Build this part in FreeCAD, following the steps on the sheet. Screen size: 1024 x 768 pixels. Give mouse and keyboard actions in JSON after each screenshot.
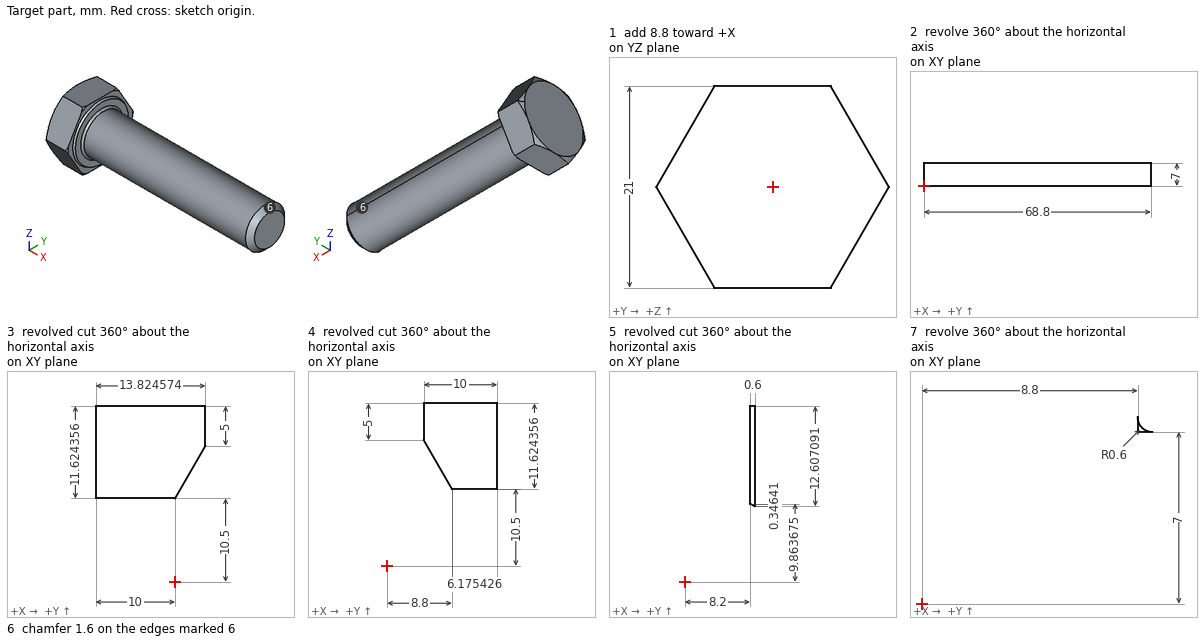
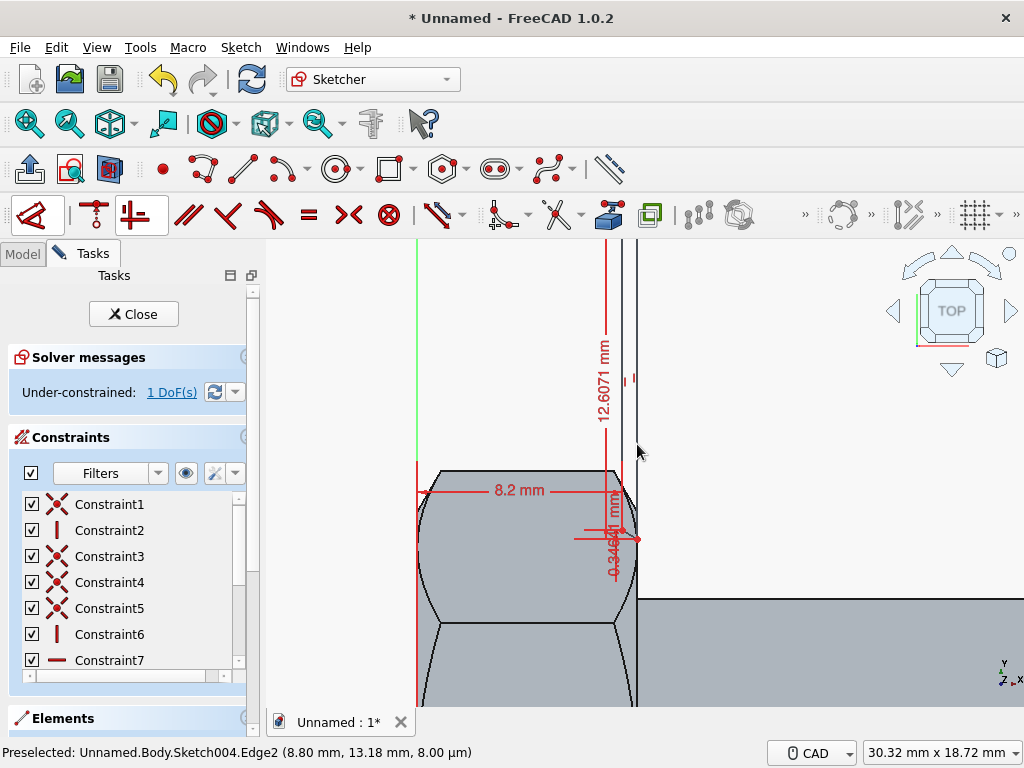
{"action": "left_click", "coordinate": [622, 530]}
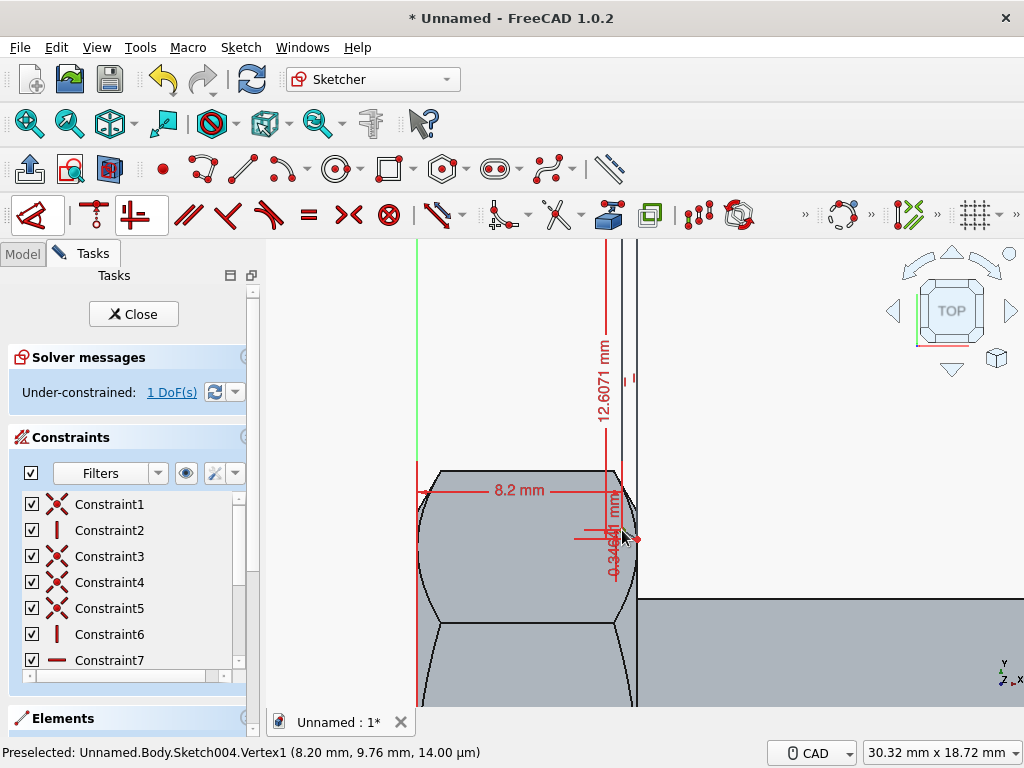
{"action": "key", "text": "i"}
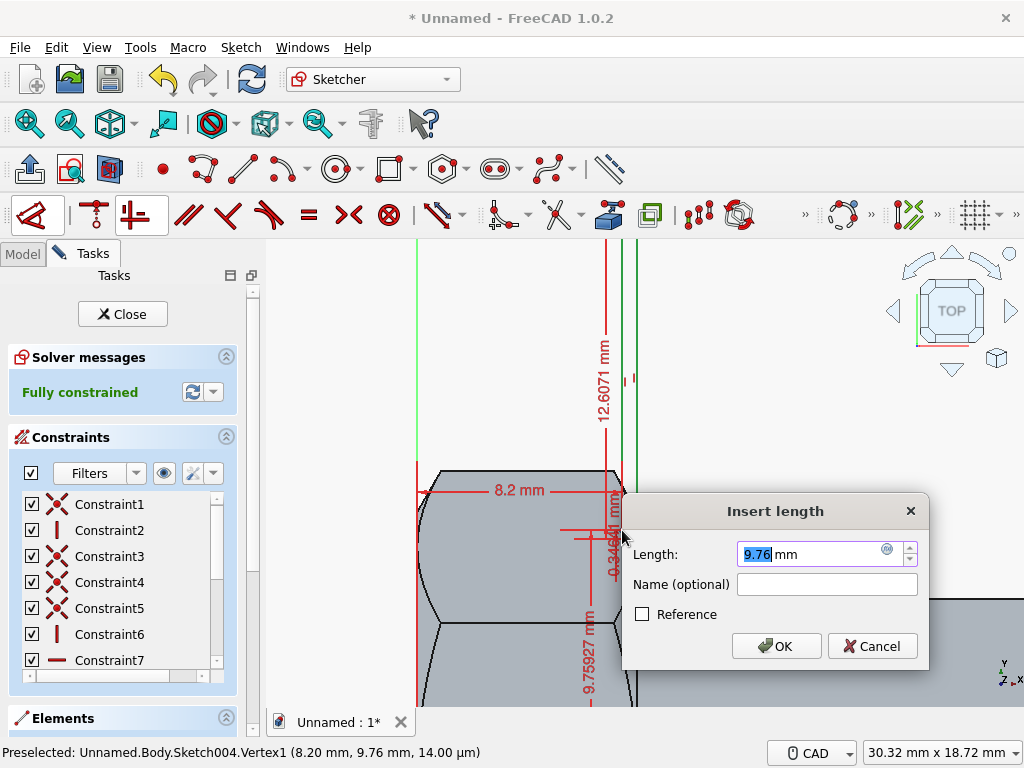
{"action": "type", "text": "9.863675"}
{"action": "key", "text": "Return"}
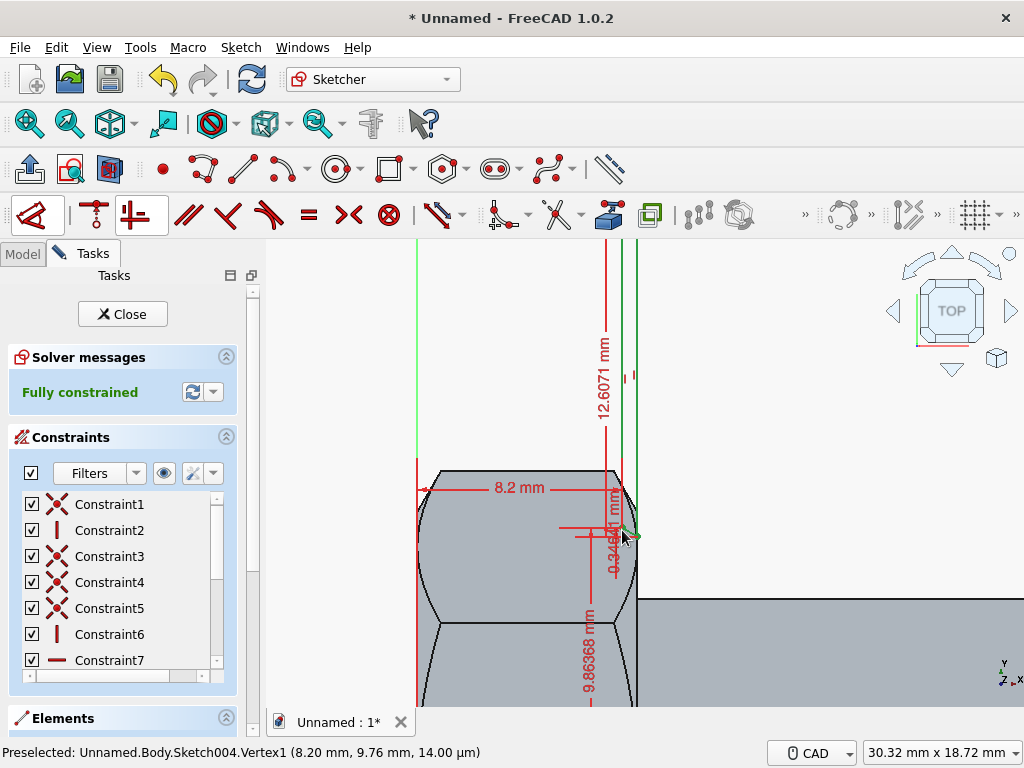
{"action": "left_click", "coordinate": [123, 314]}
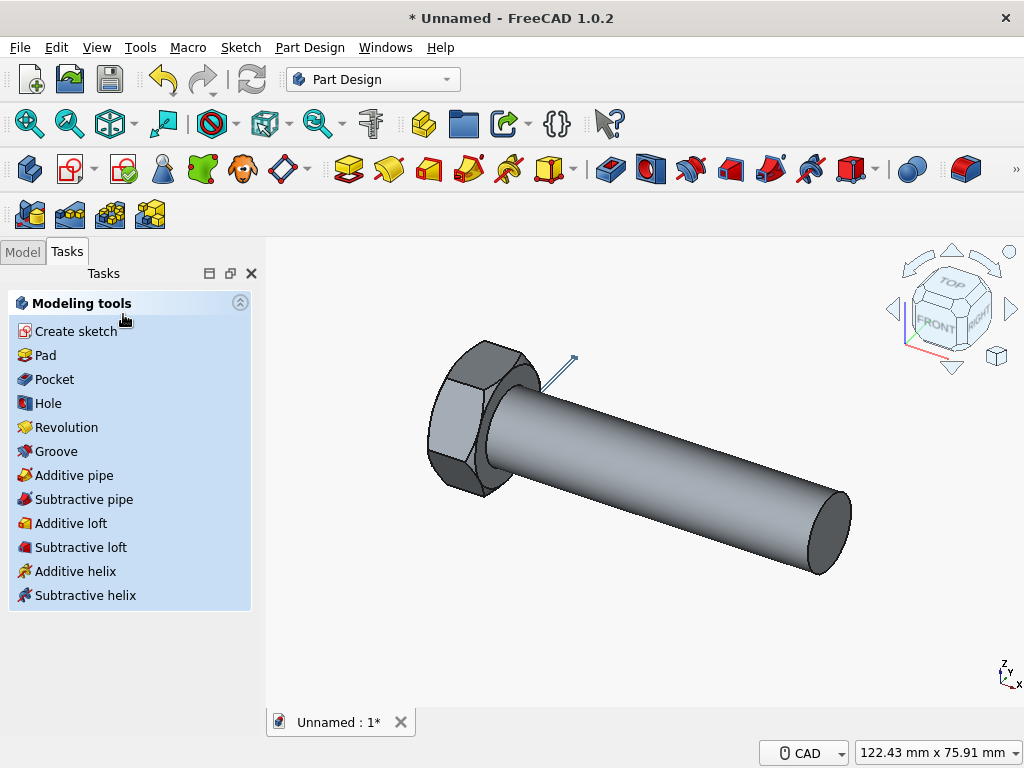
{"action": "left_click", "coordinate": [692, 170]}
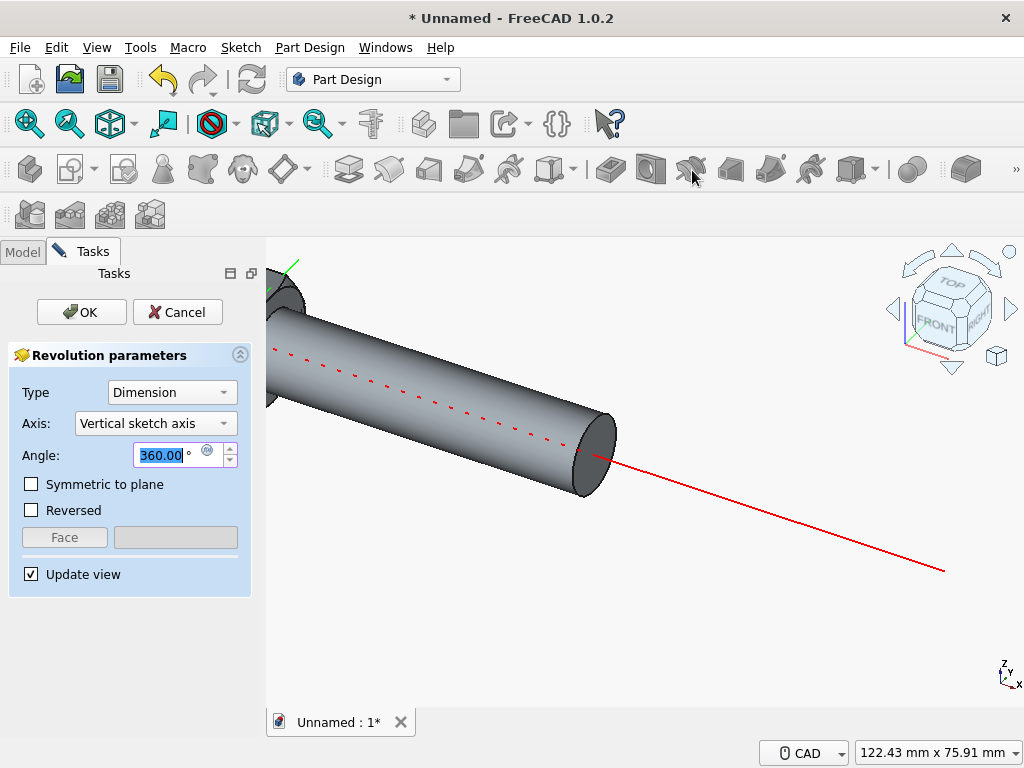
{"action": "left_click", "coordinate": [156, 424]}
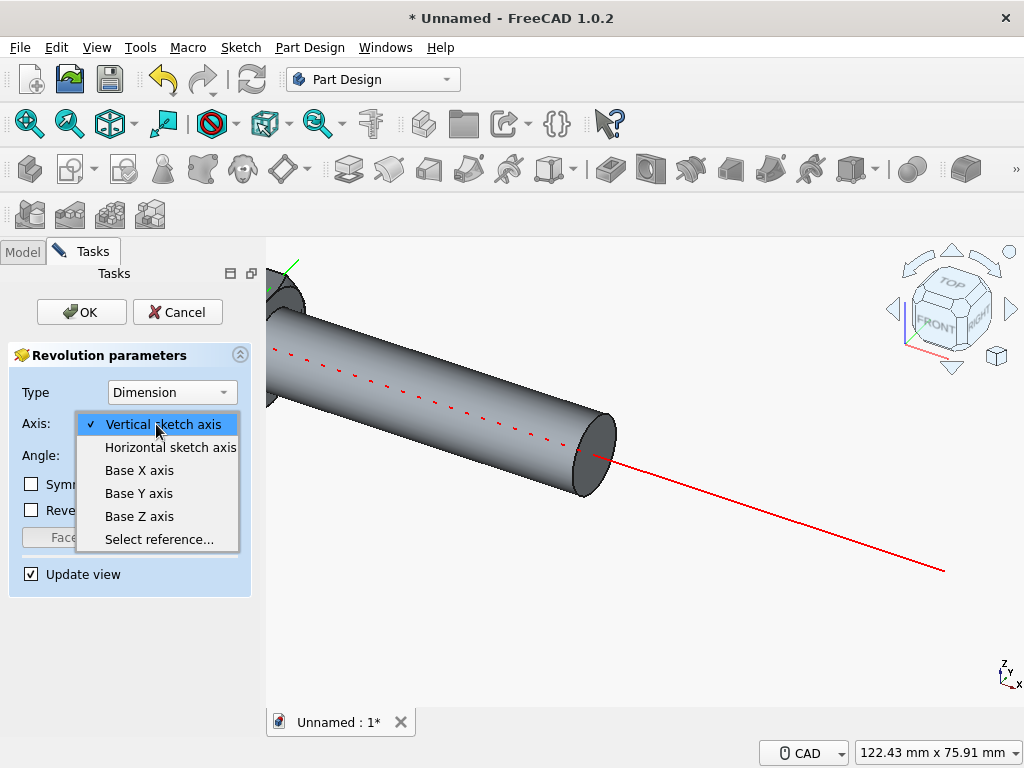
{"action": "left_click", "coordinate": [156, 448]}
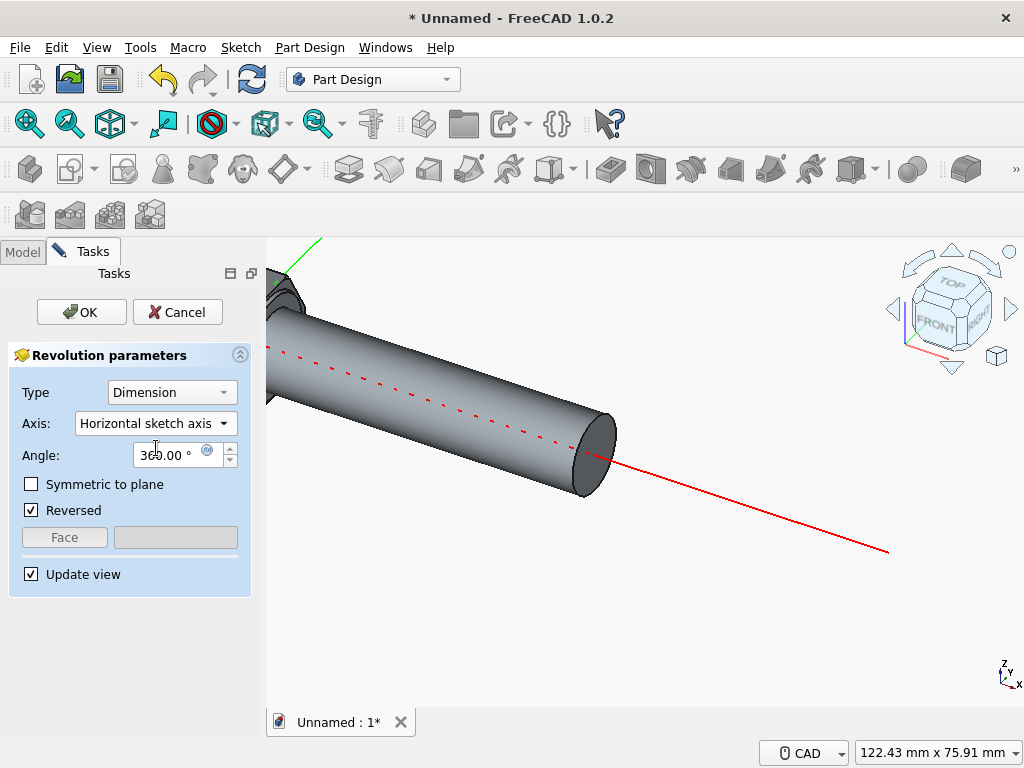
{"action": "left_click", "coordinate": [82, 312]}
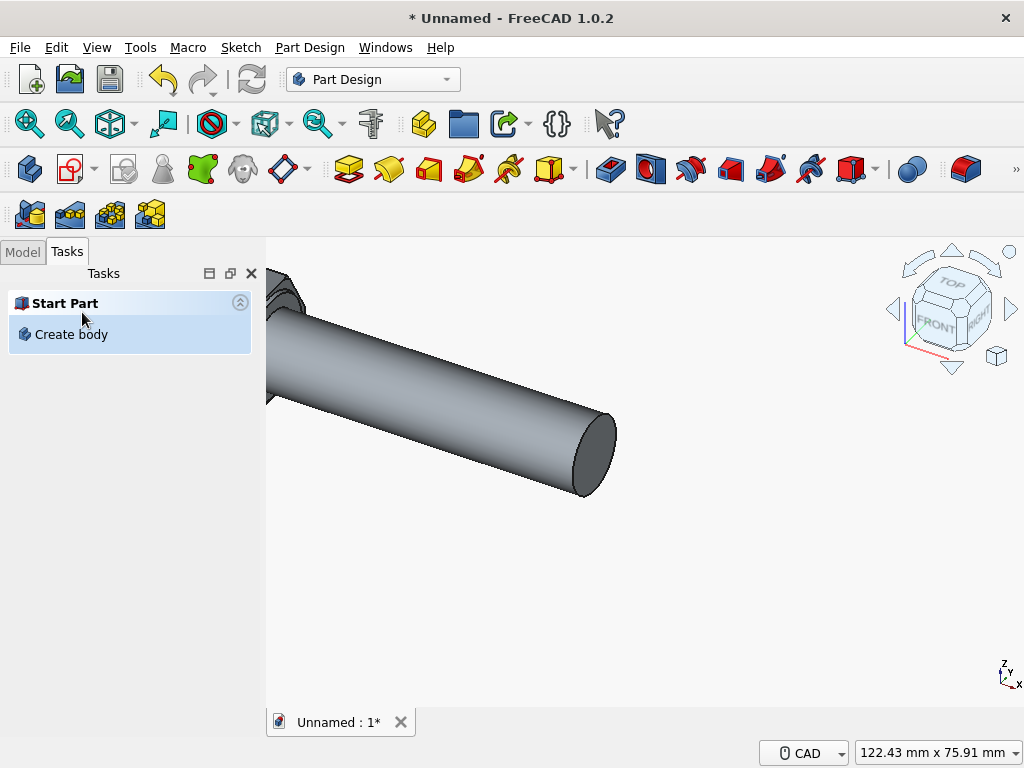
{"action": "key", "text": "v f"}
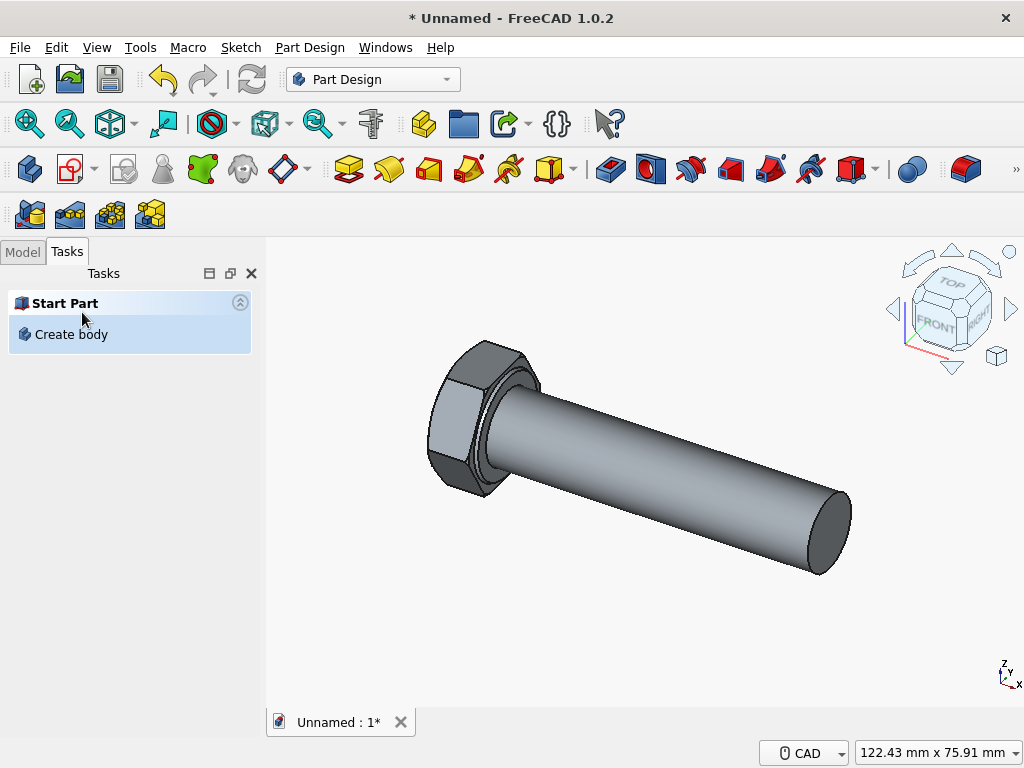
{"action": "left_click", "coordinate": [808, 554]}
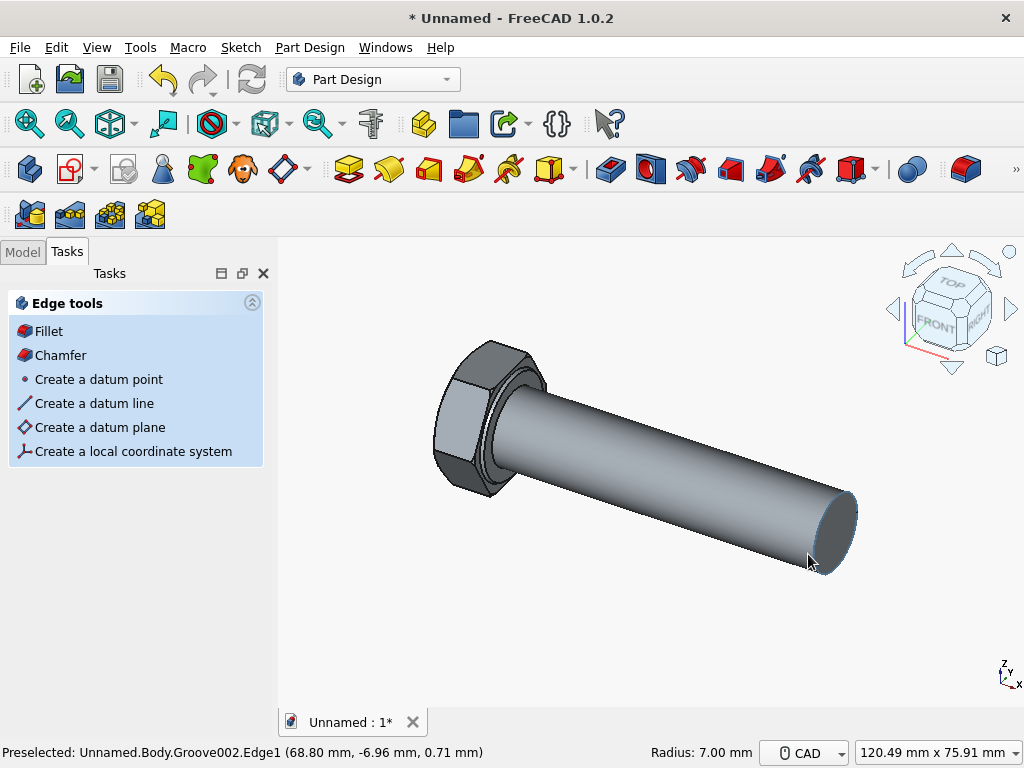
{"action": "left_click", "coordinate": [136, 355]}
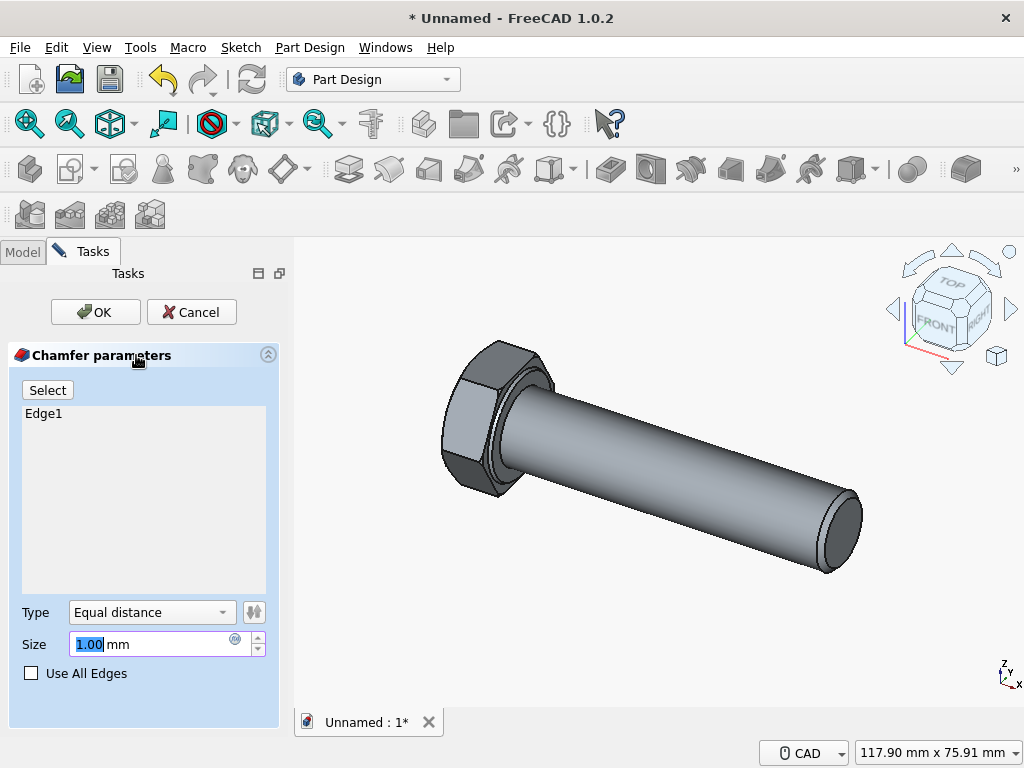
{"action": "type", "text": "1.6"}
{"action": "key", "text": "Tab"}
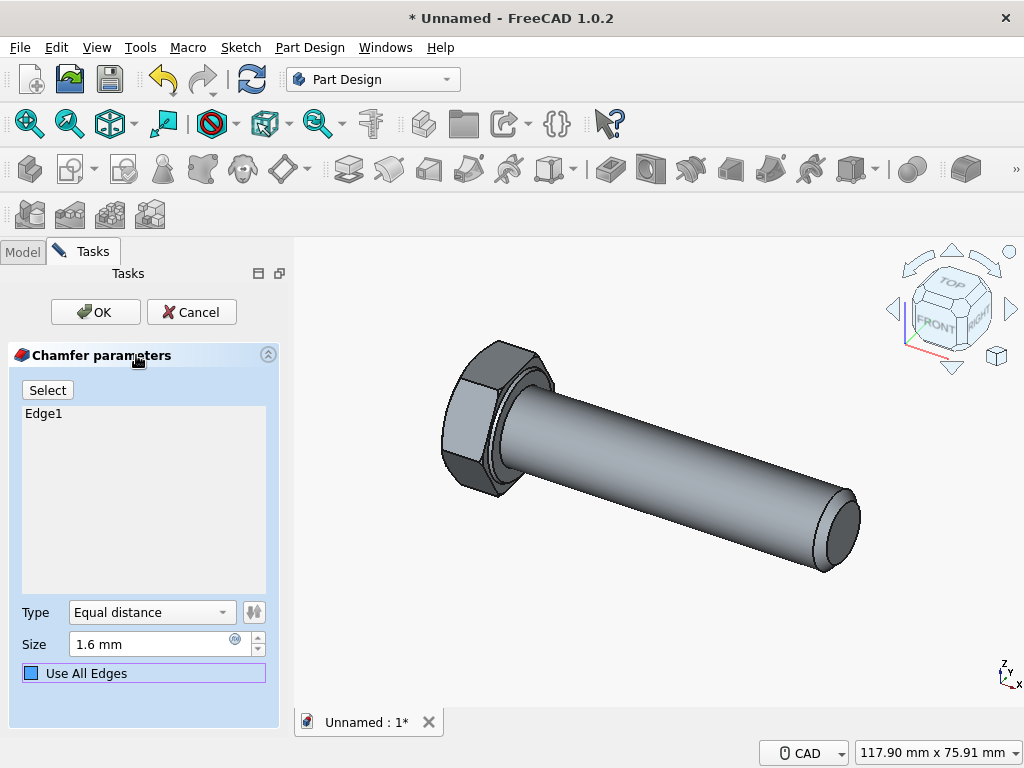
{"action": "left_click", "coordinate": [96, 312]}